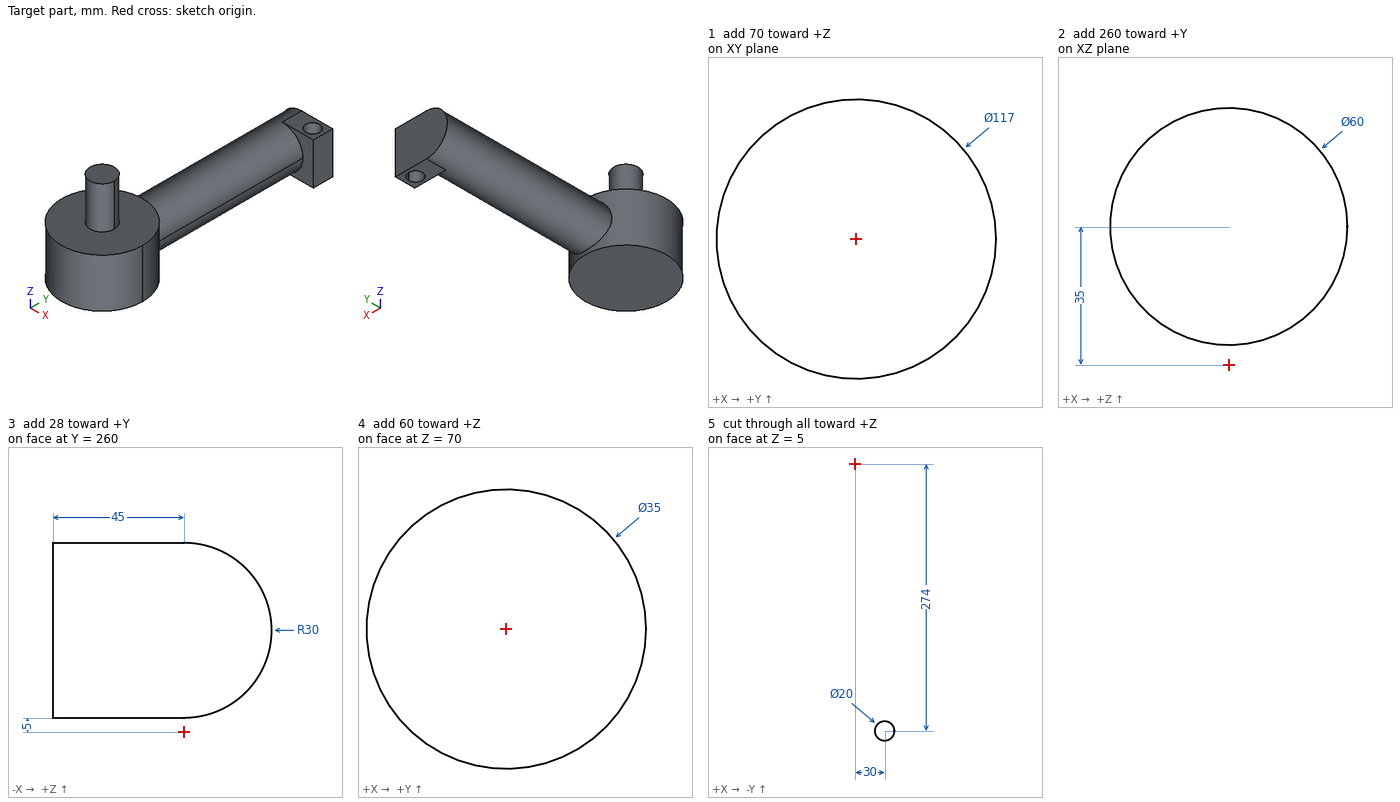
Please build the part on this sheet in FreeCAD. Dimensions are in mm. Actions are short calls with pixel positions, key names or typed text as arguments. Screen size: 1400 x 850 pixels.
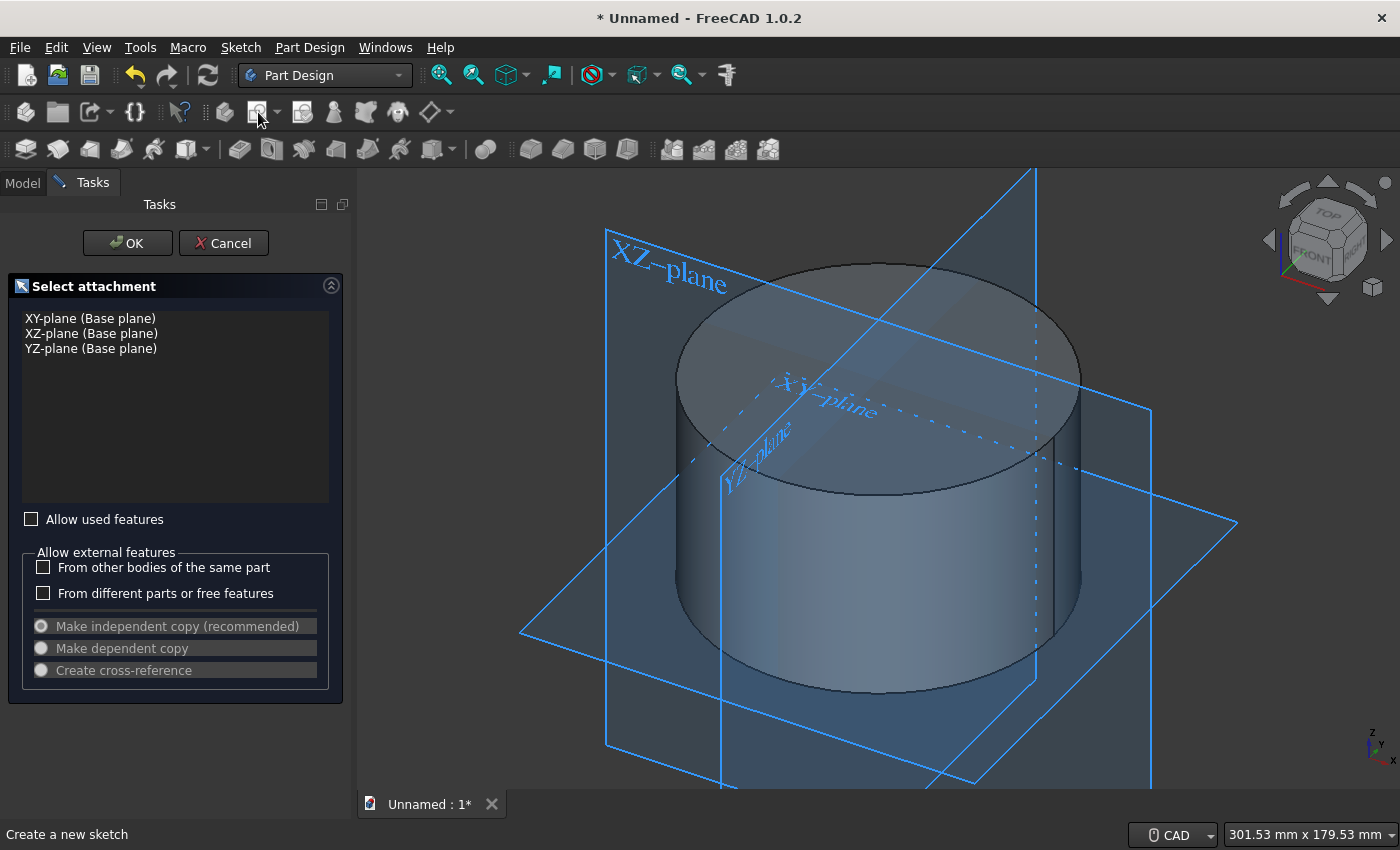
click(82, 334)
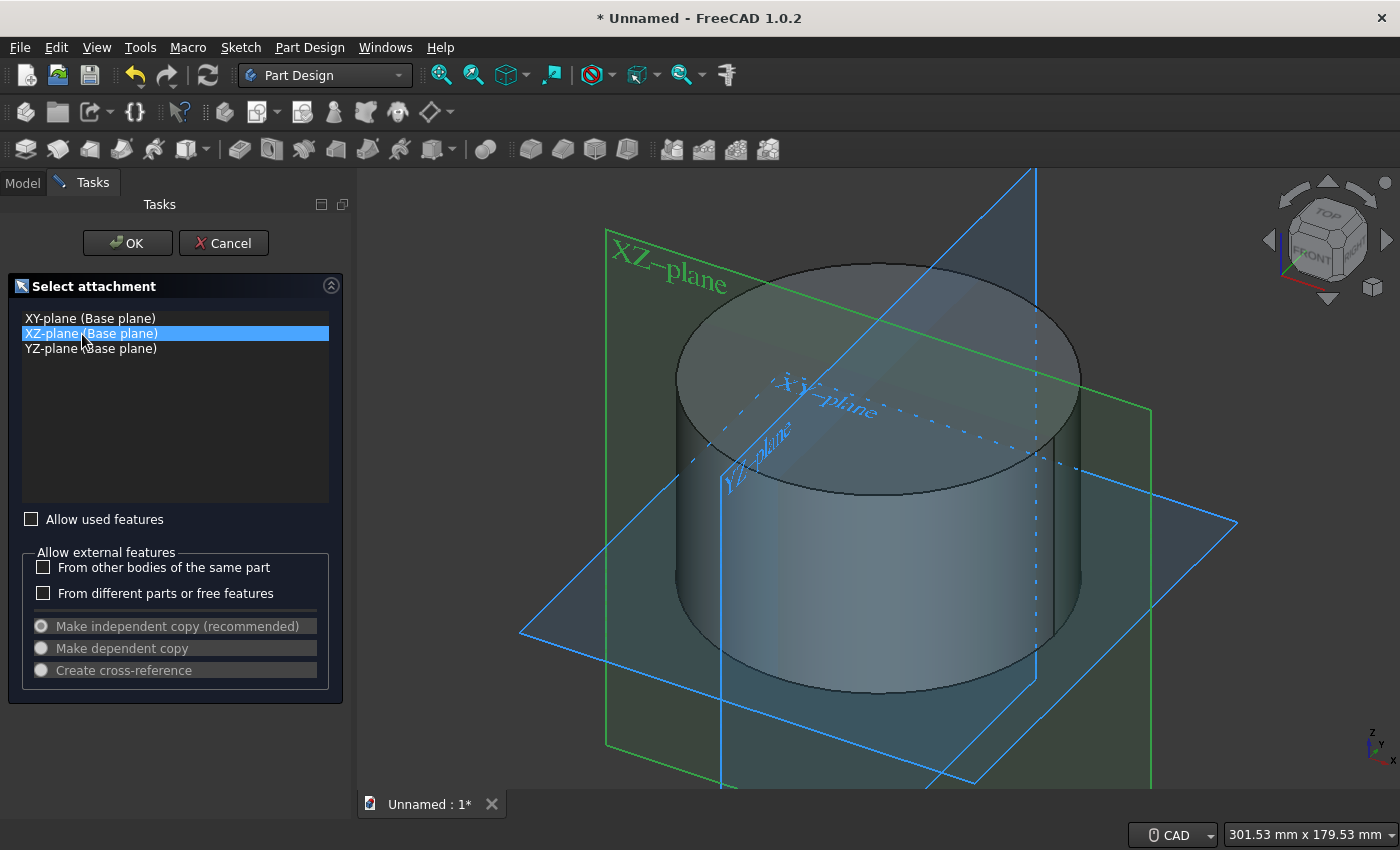
click(128, 243)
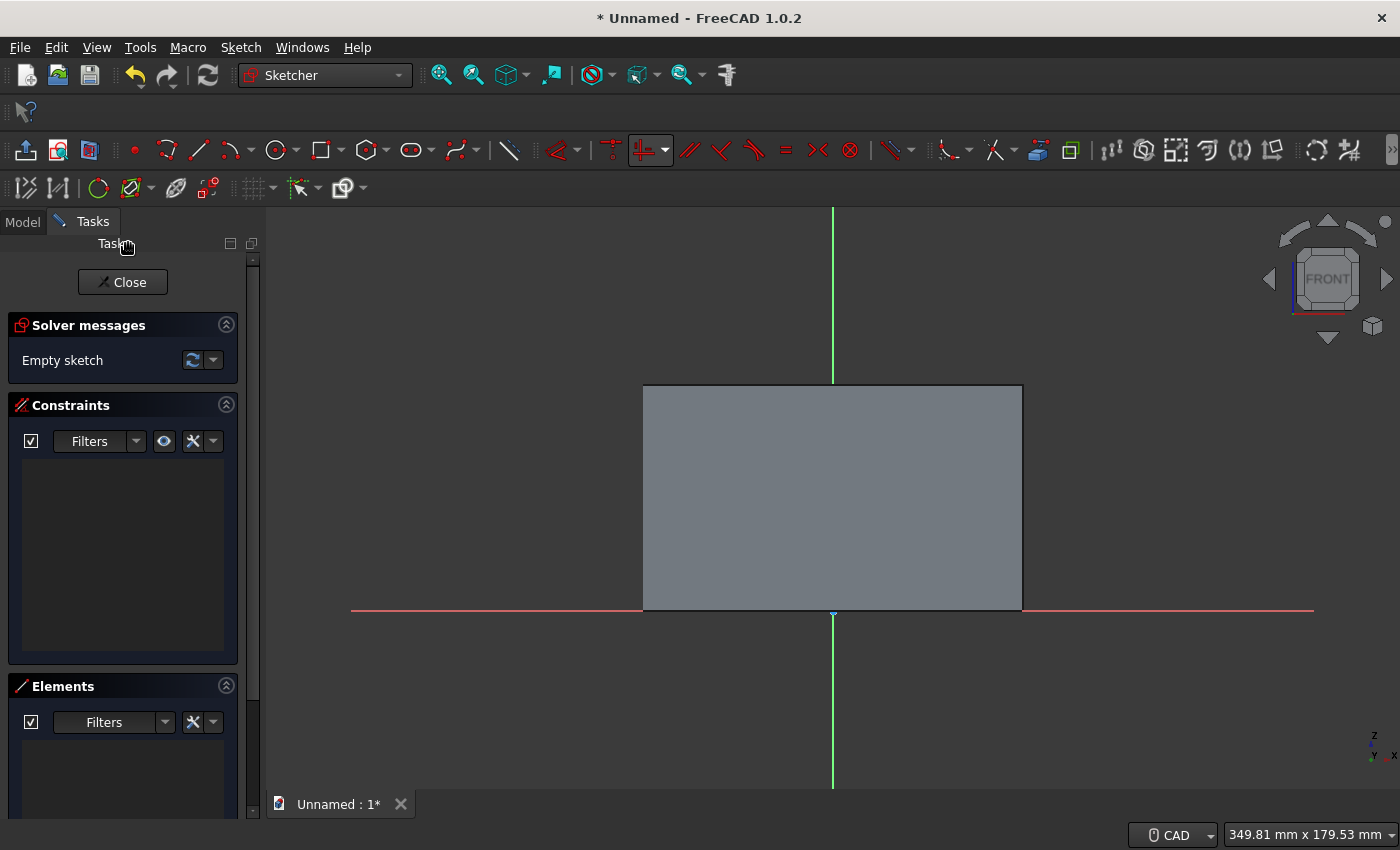
key(q)
key(s)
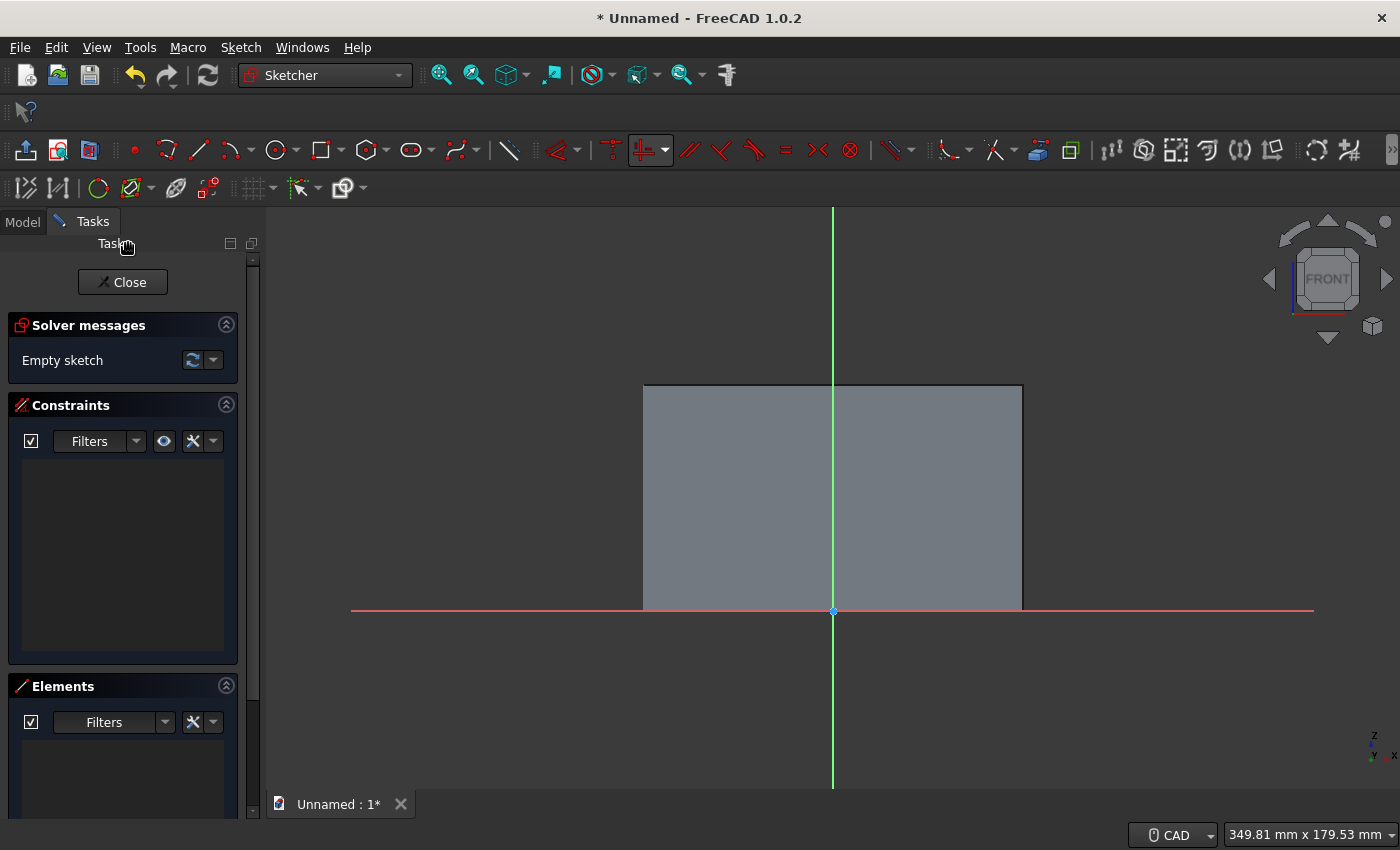
scroll(916, 516, up, 3)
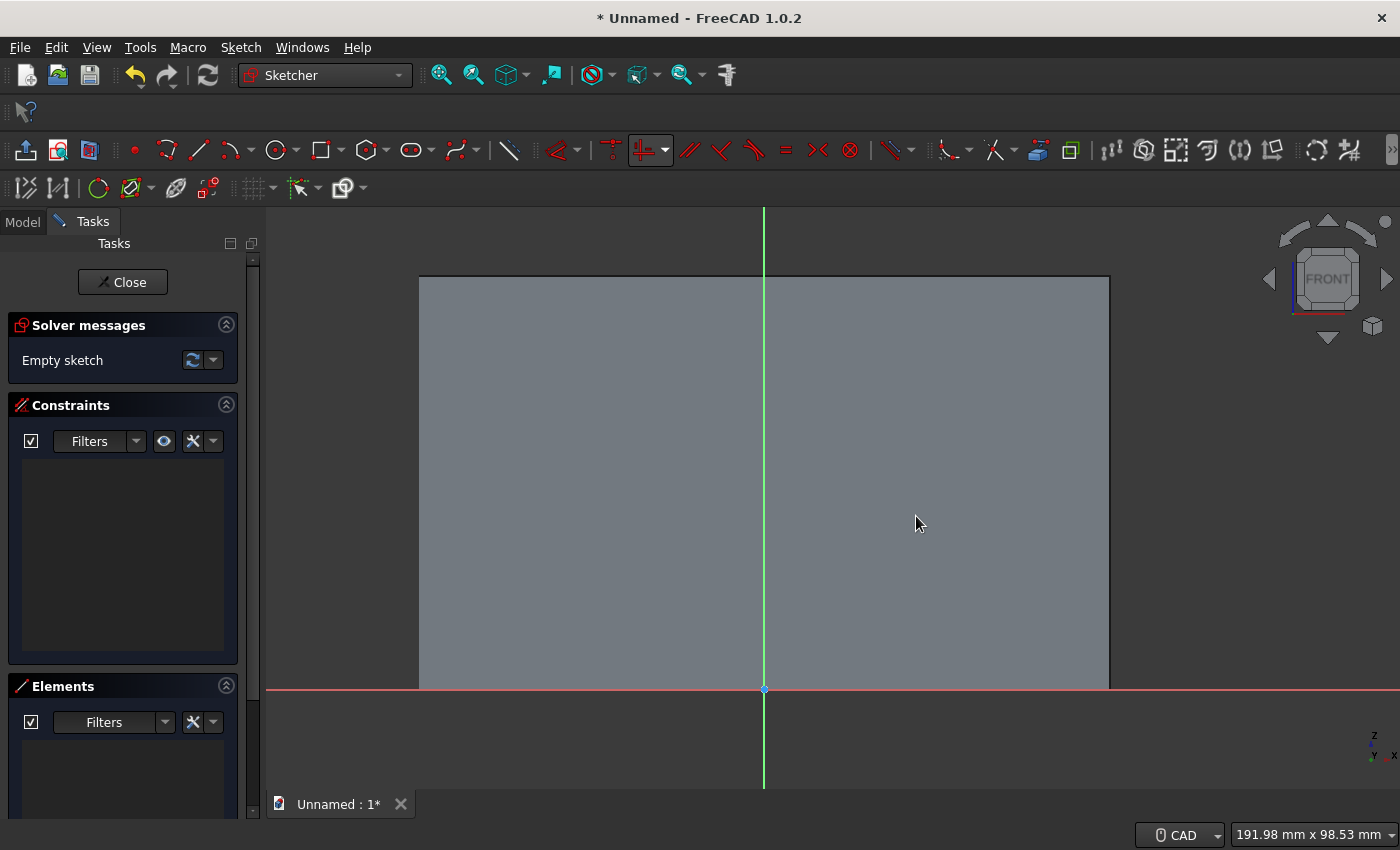
click(276, 150)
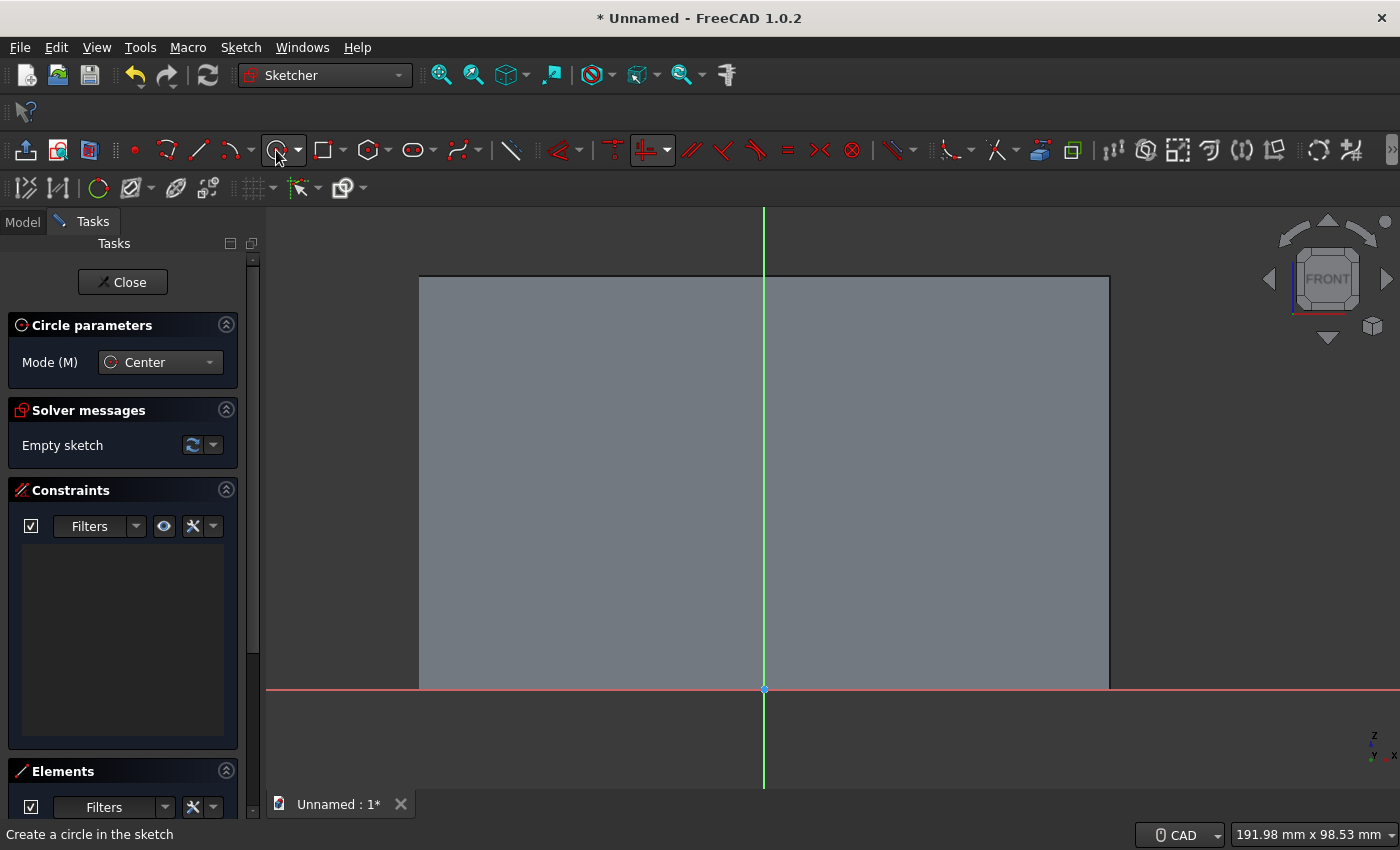
click(764, 483)
click(890, 357)
key(Escape)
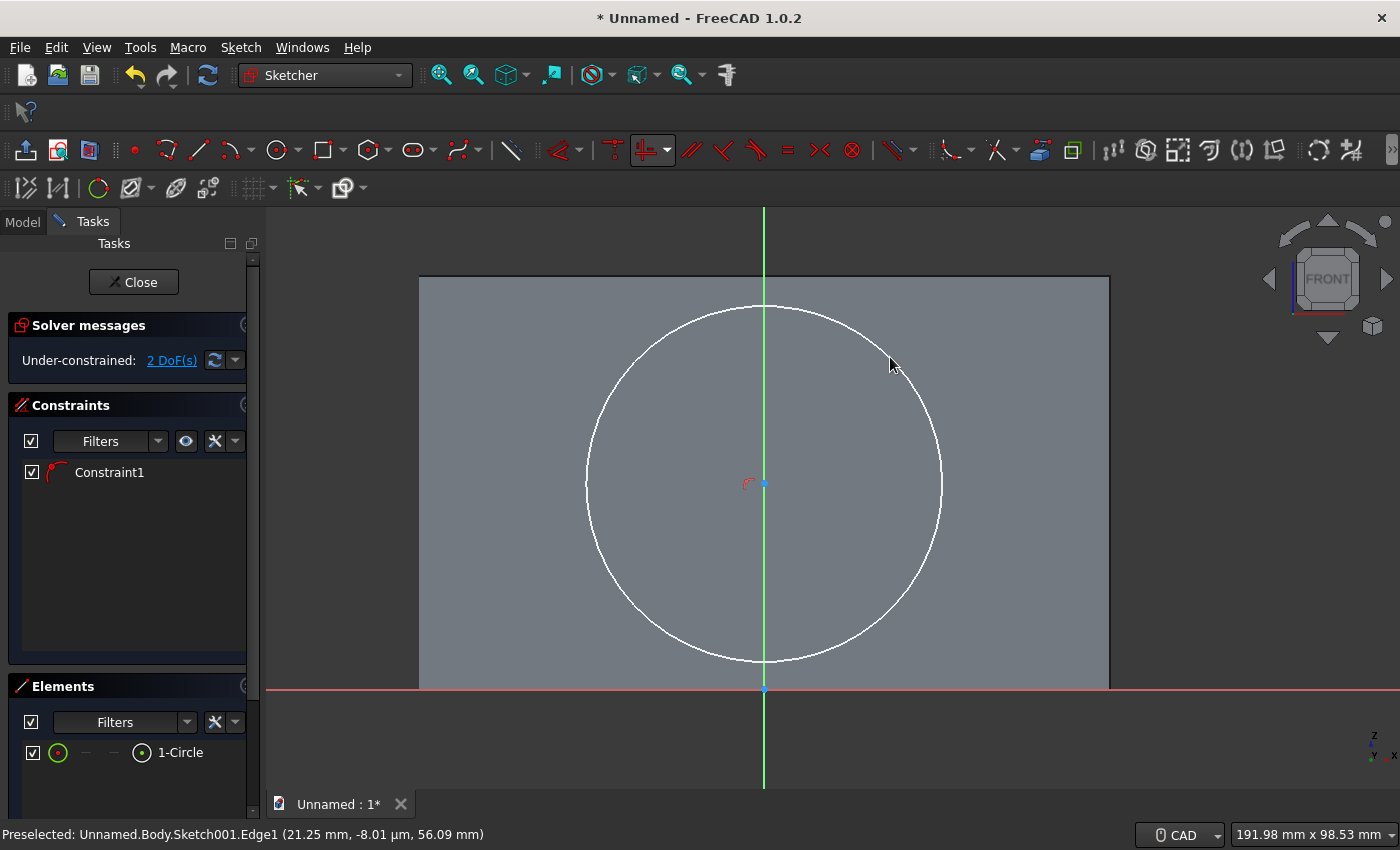
key(d)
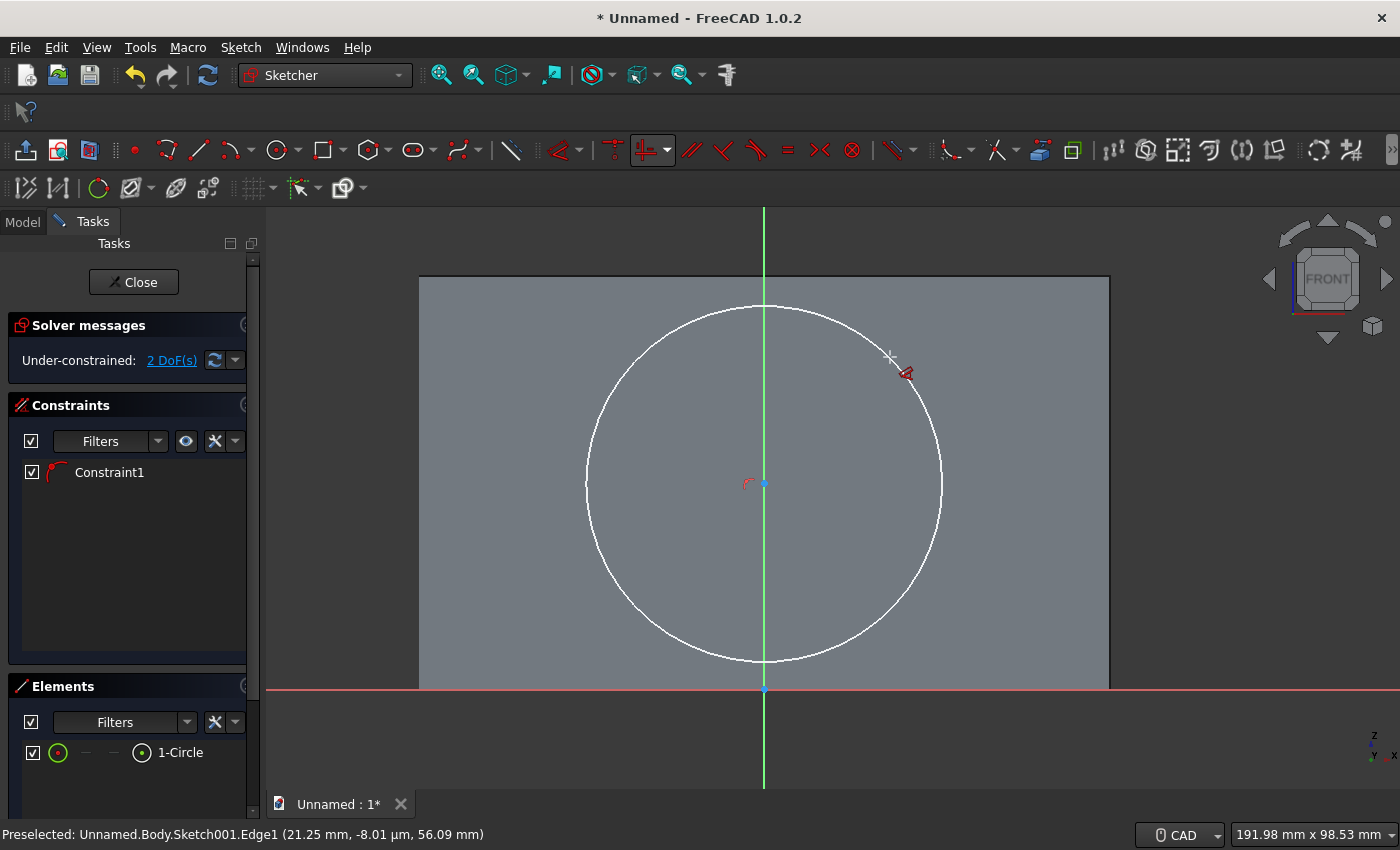
click(890, 358)
click(913, 335)